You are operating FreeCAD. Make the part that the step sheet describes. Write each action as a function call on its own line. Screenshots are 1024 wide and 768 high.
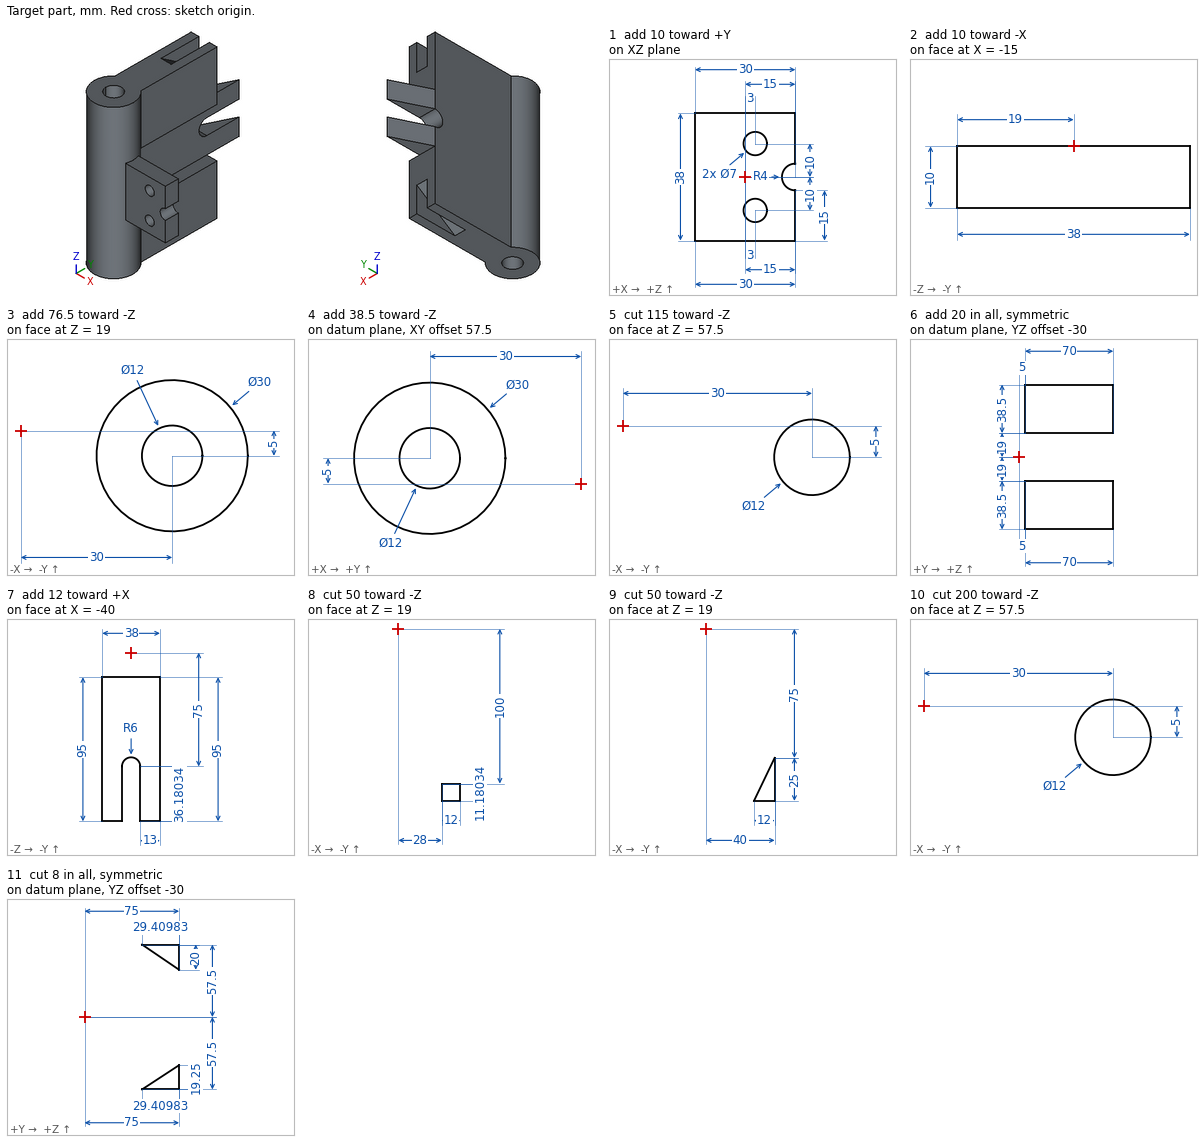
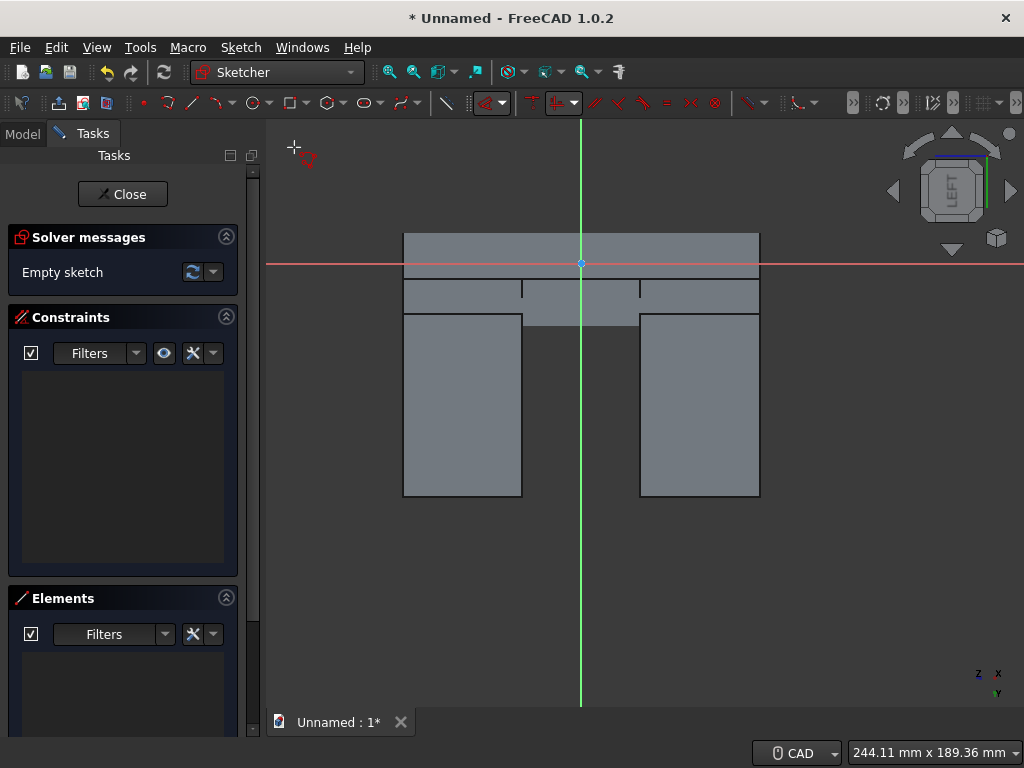
click(600, 497)
click(600, 609)
click(640, 609)
click(640, 314)
click(522, 314)
click(522, 609)
click(563, 609)
click(563, 497)
right_click(563, 497)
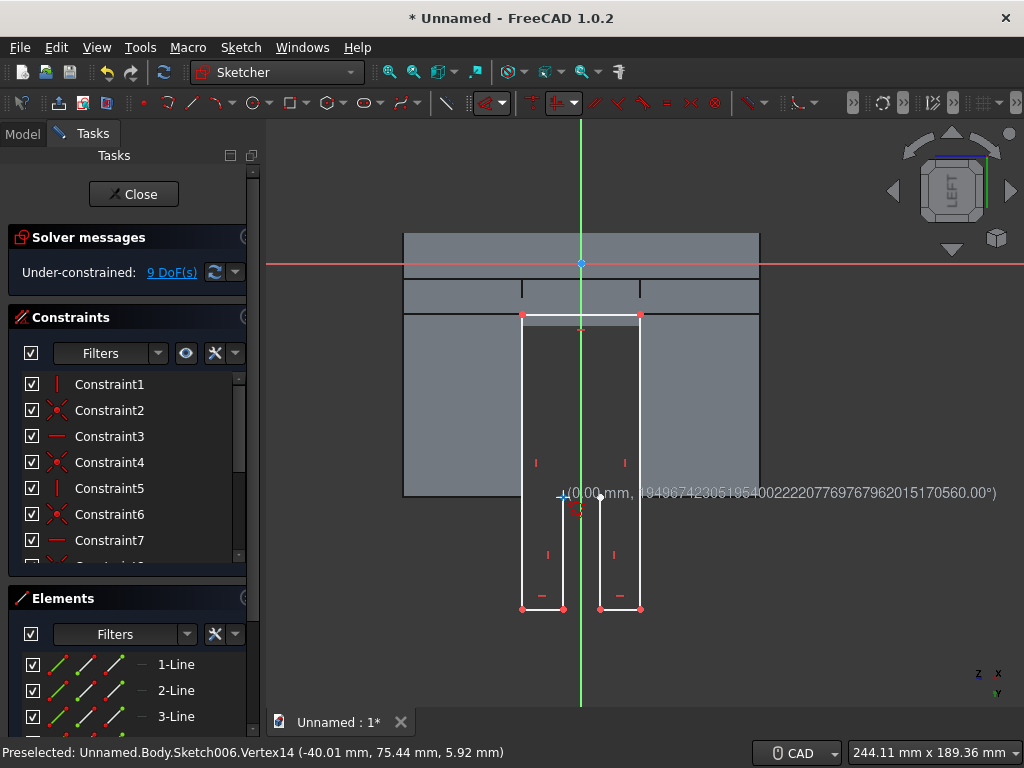
click(216, 104)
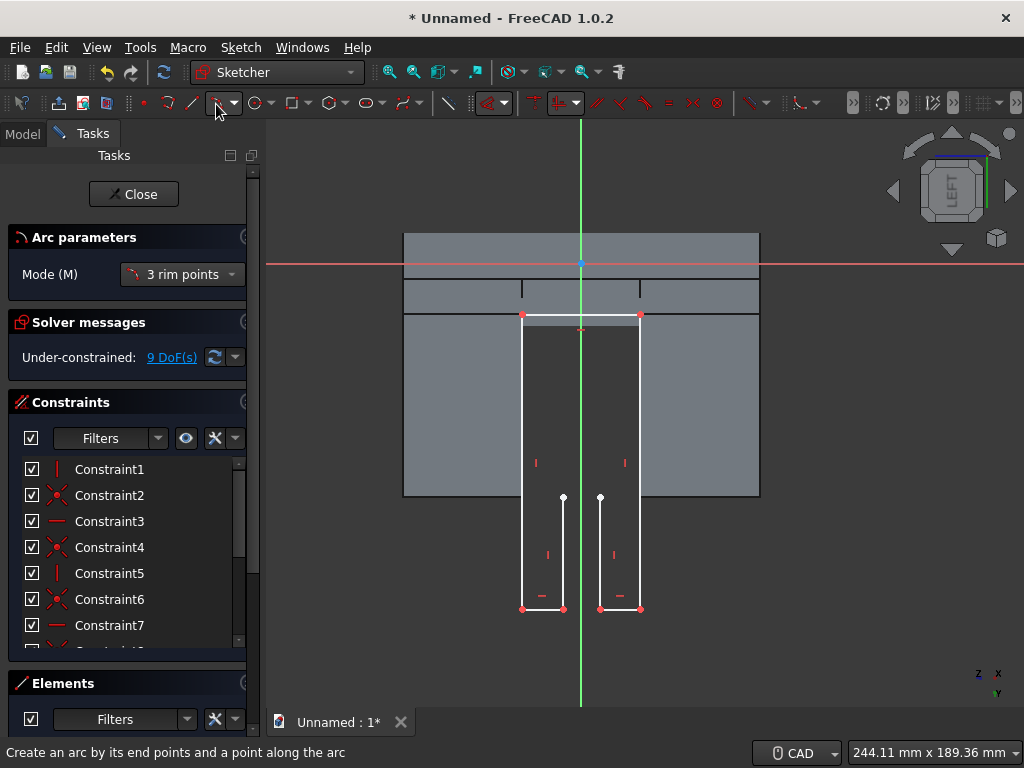
click(563, 498)
click(600, 498)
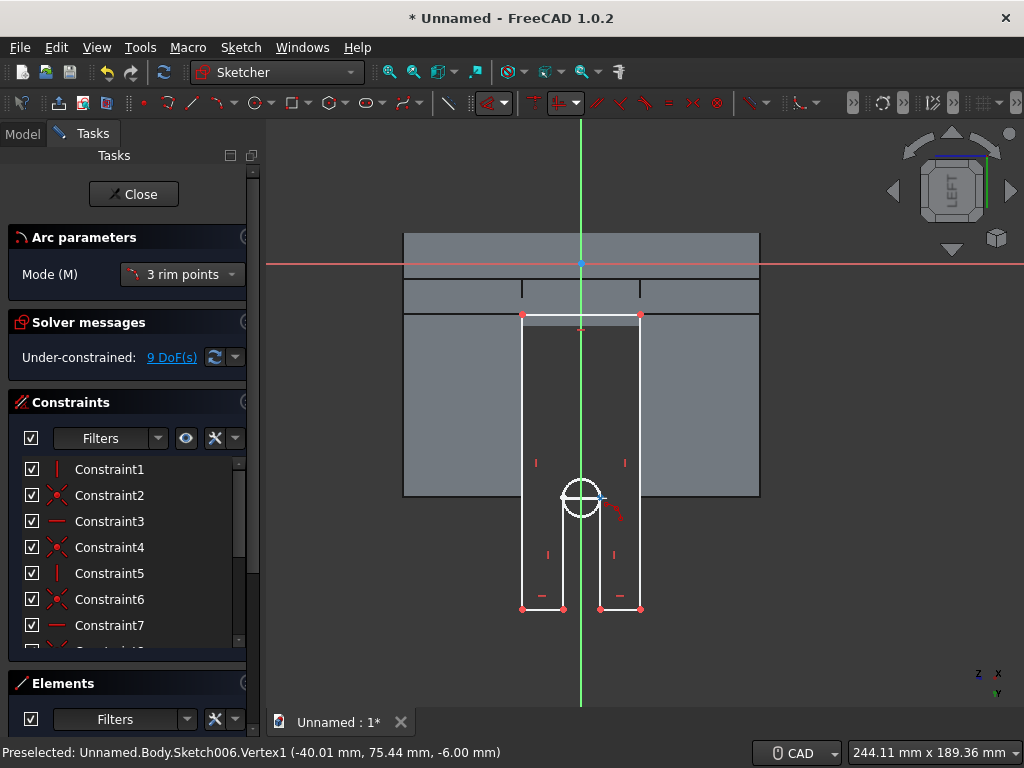
scroll(592, 482, up, 2)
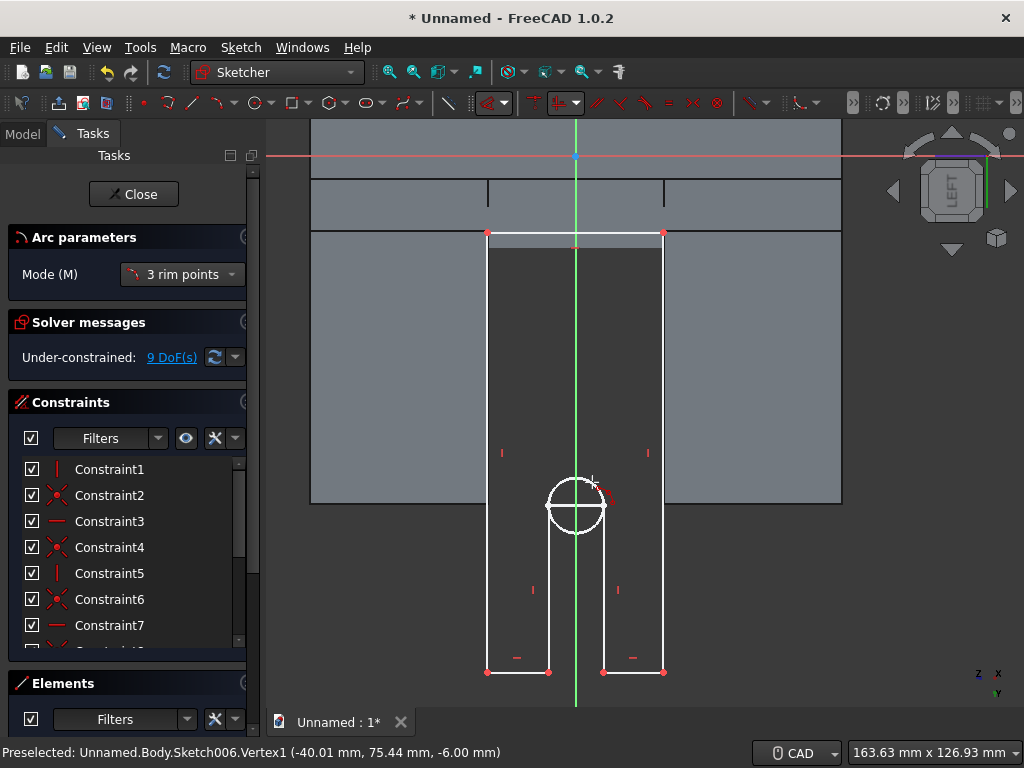
click(592, 481)
key(Escape)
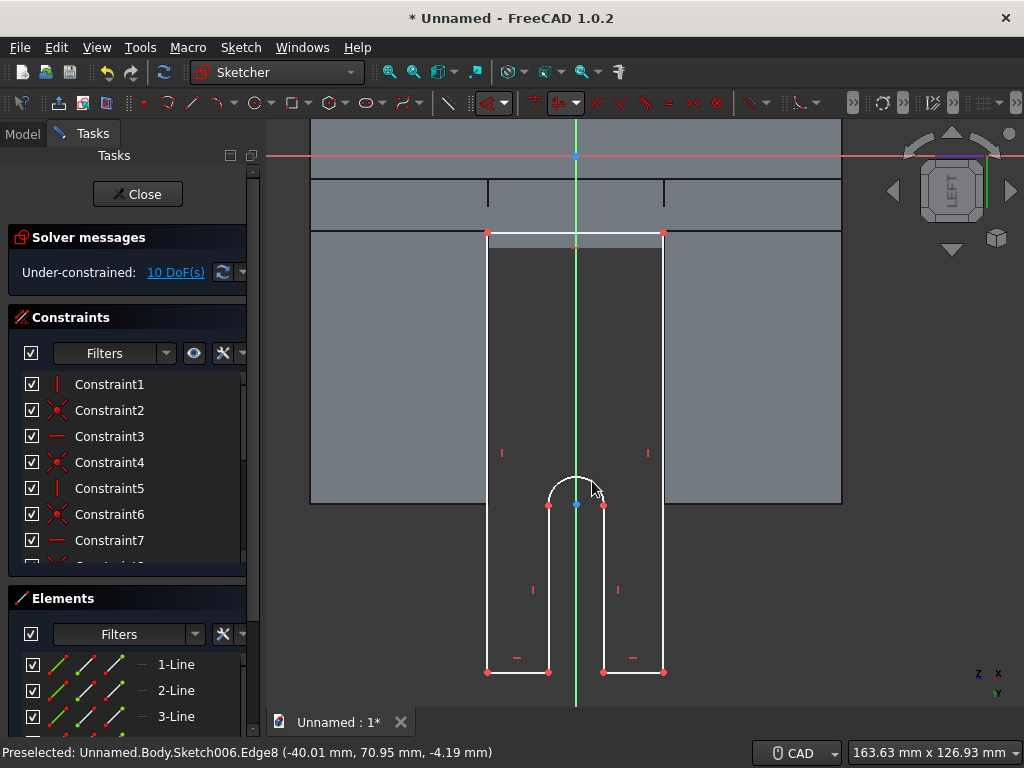
click(604, 556)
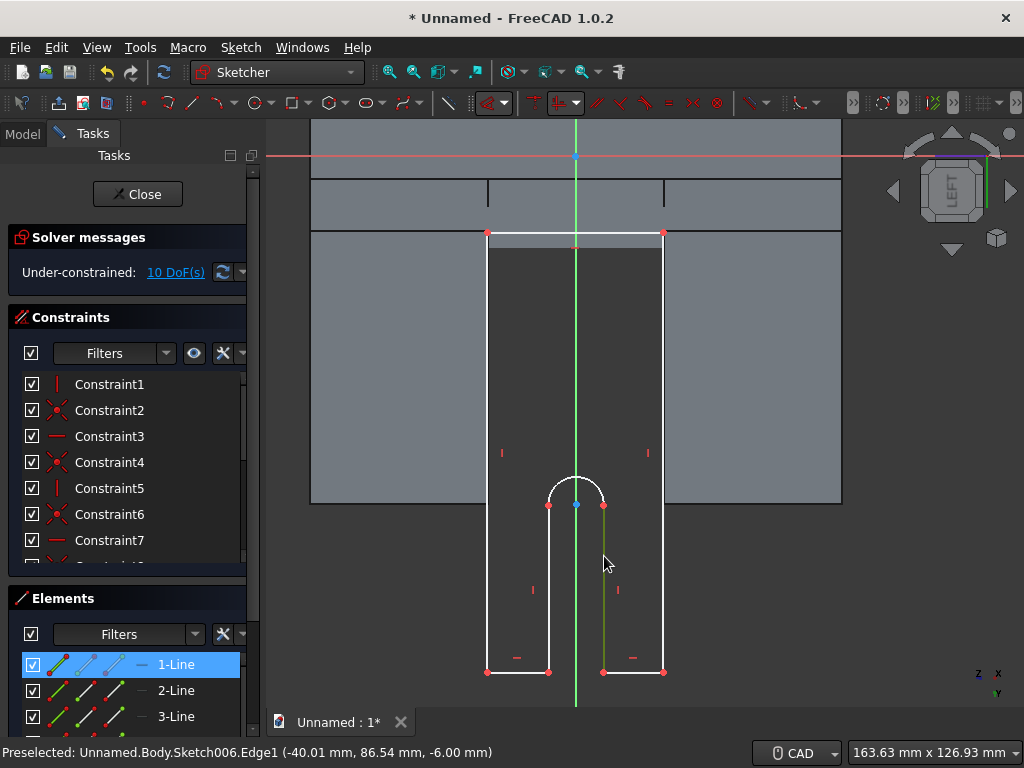
click(593, 482)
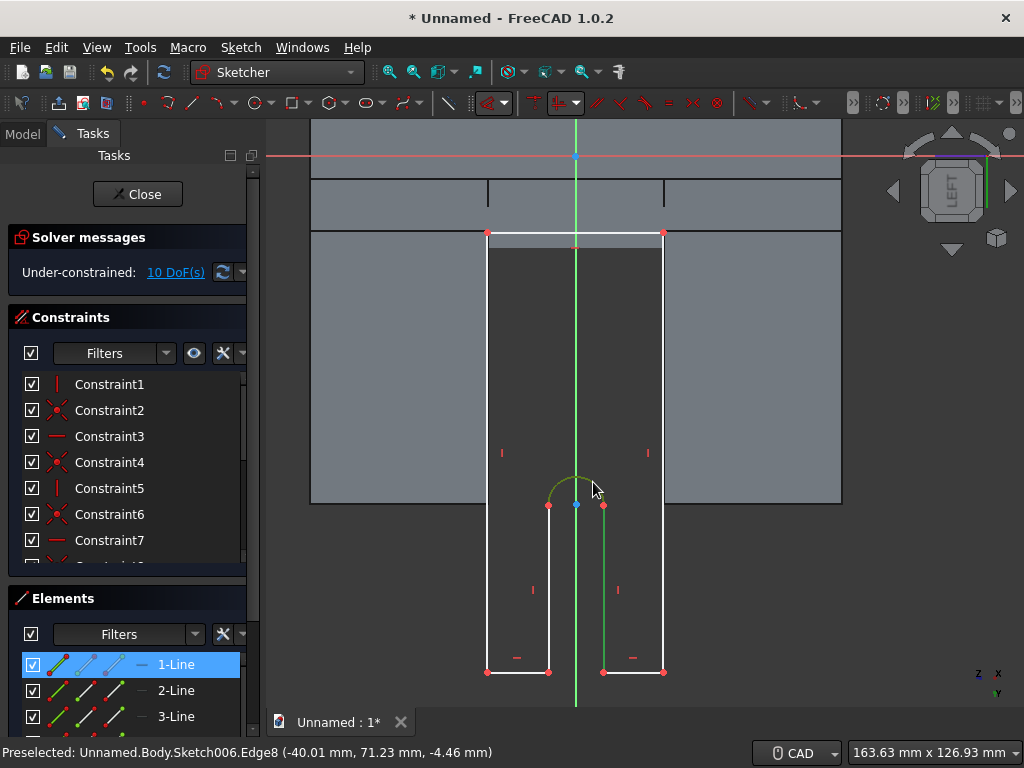
key(t)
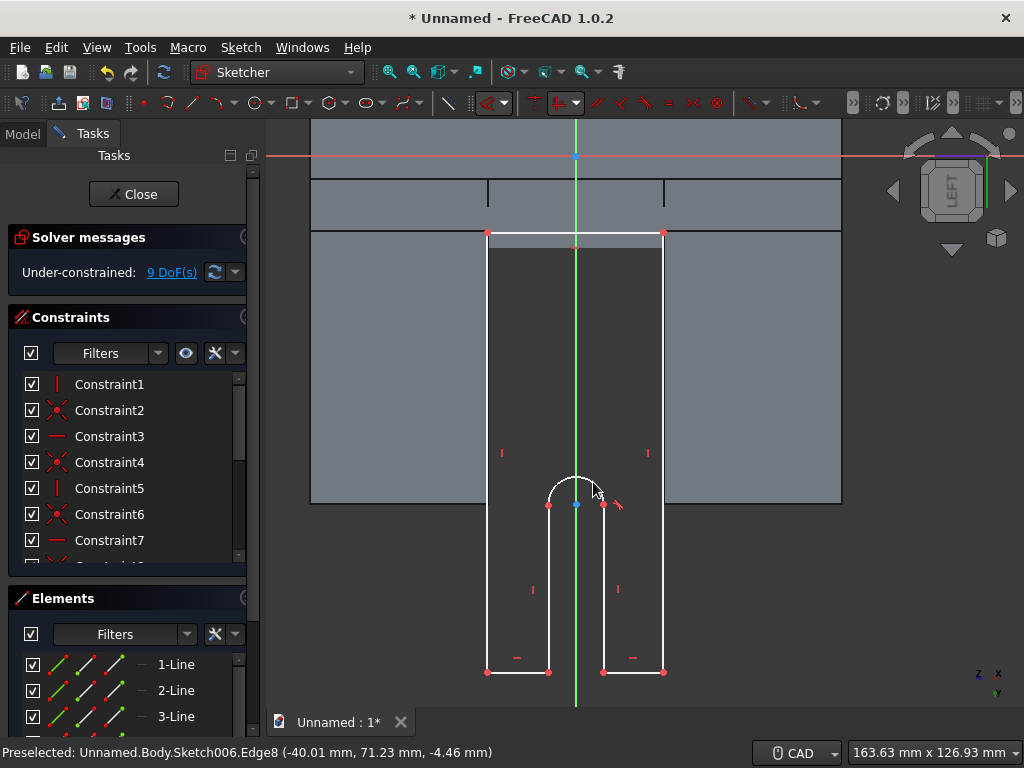
click(549, 623)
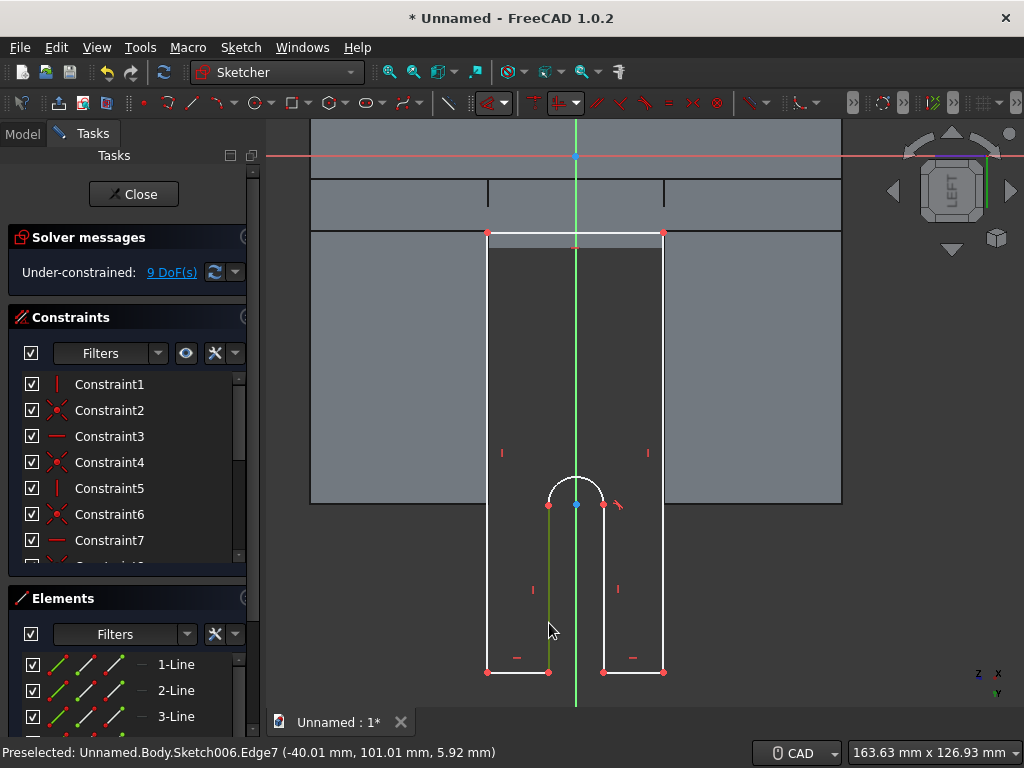
click(592, 482)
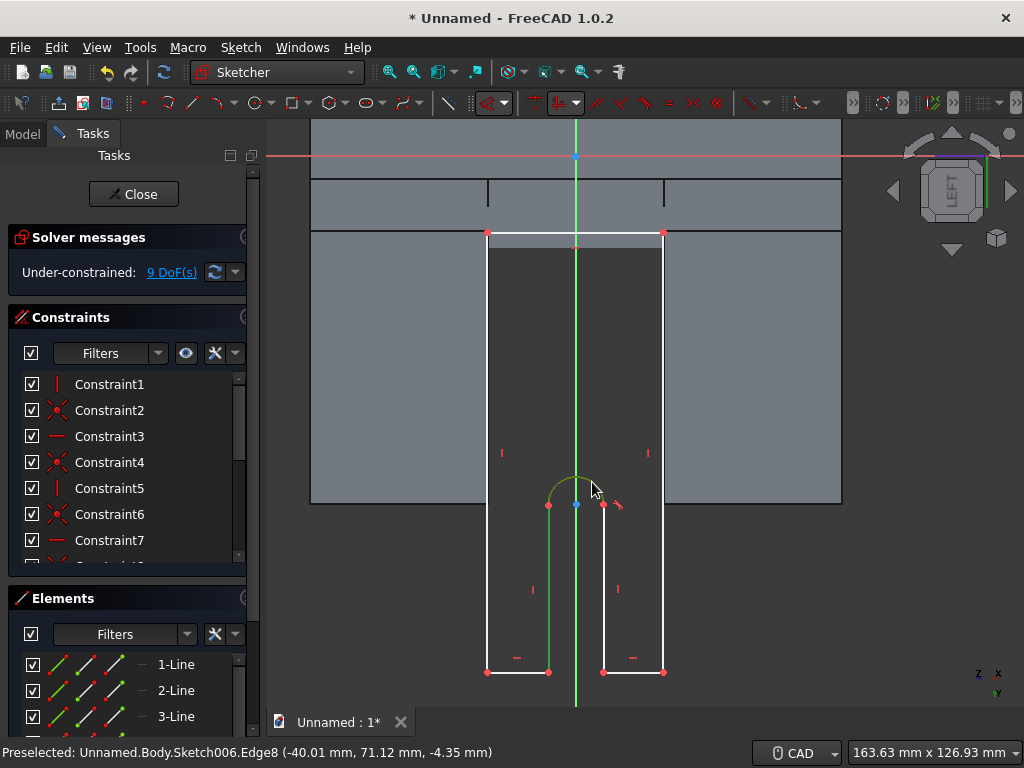
click(646, 104)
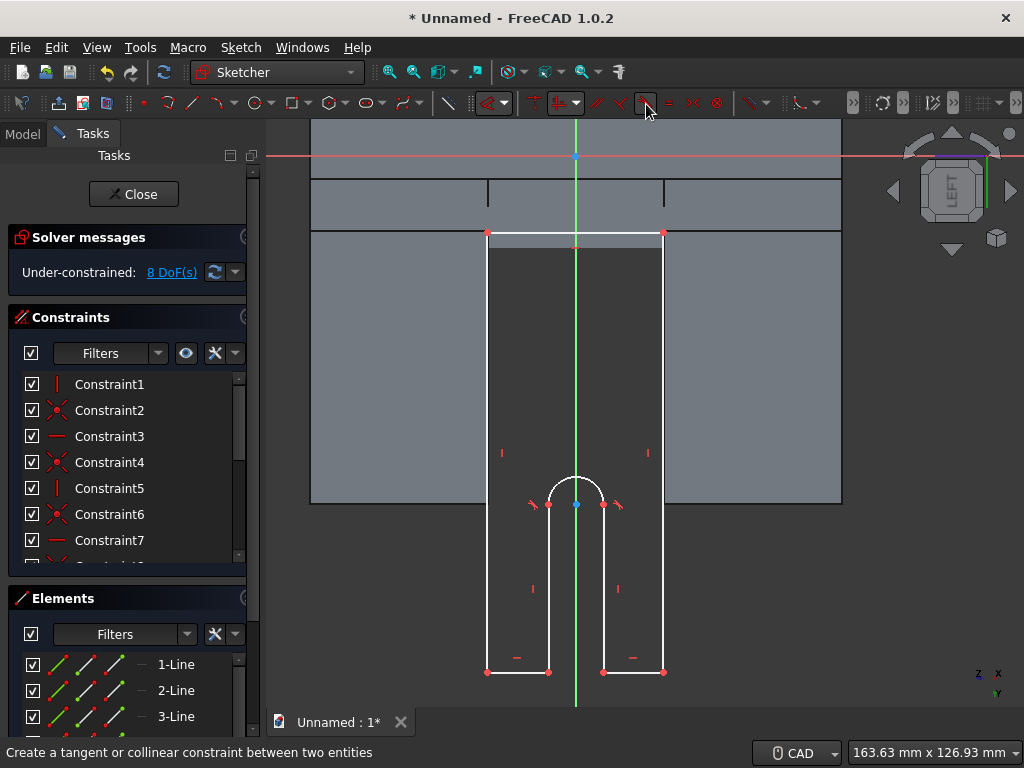
click(576, 505)